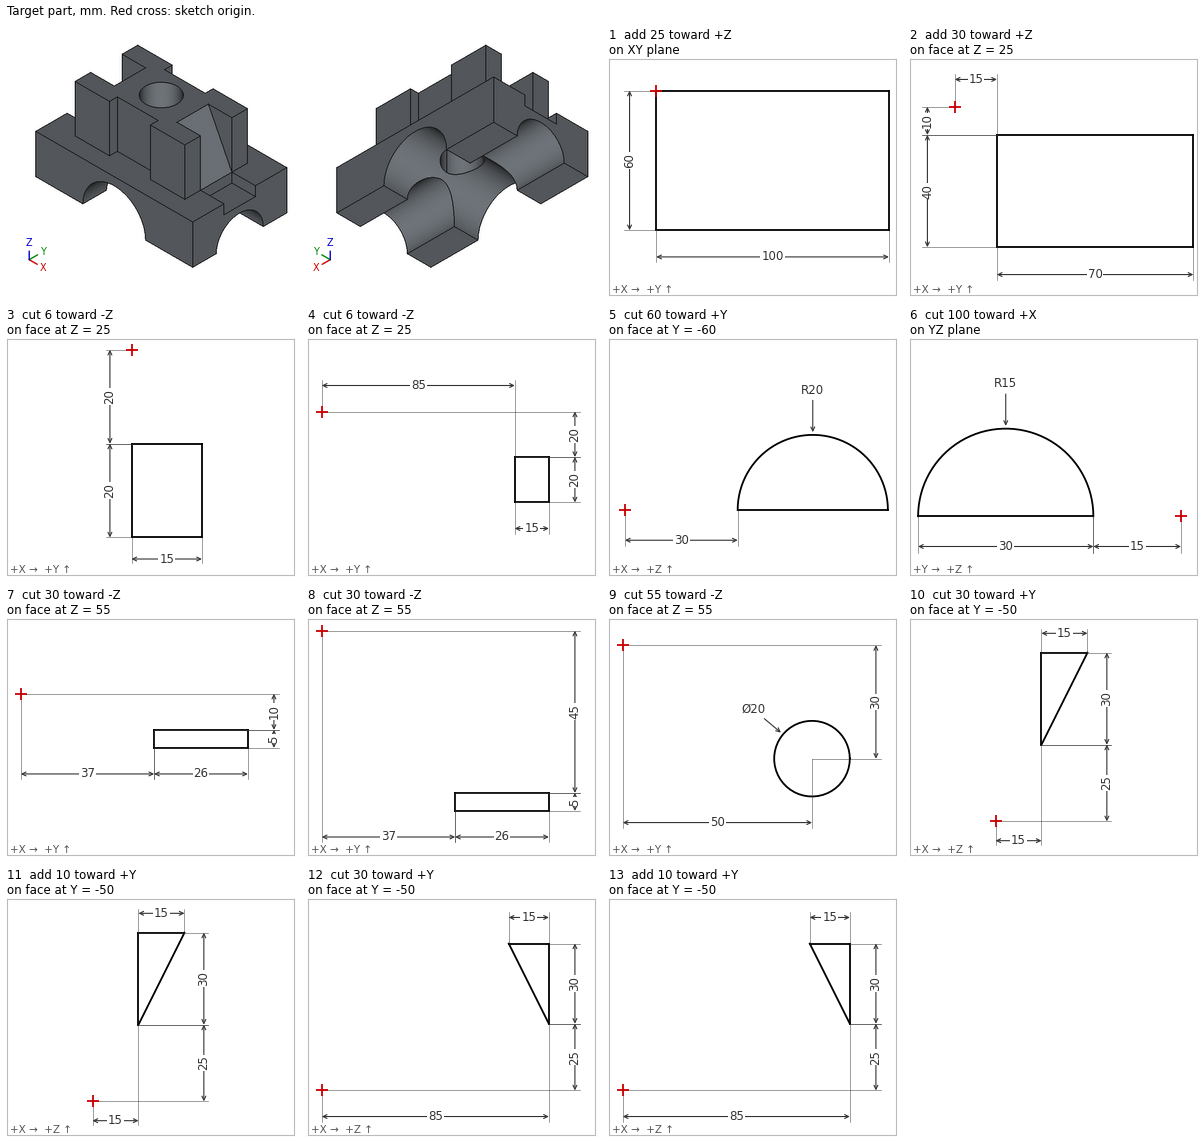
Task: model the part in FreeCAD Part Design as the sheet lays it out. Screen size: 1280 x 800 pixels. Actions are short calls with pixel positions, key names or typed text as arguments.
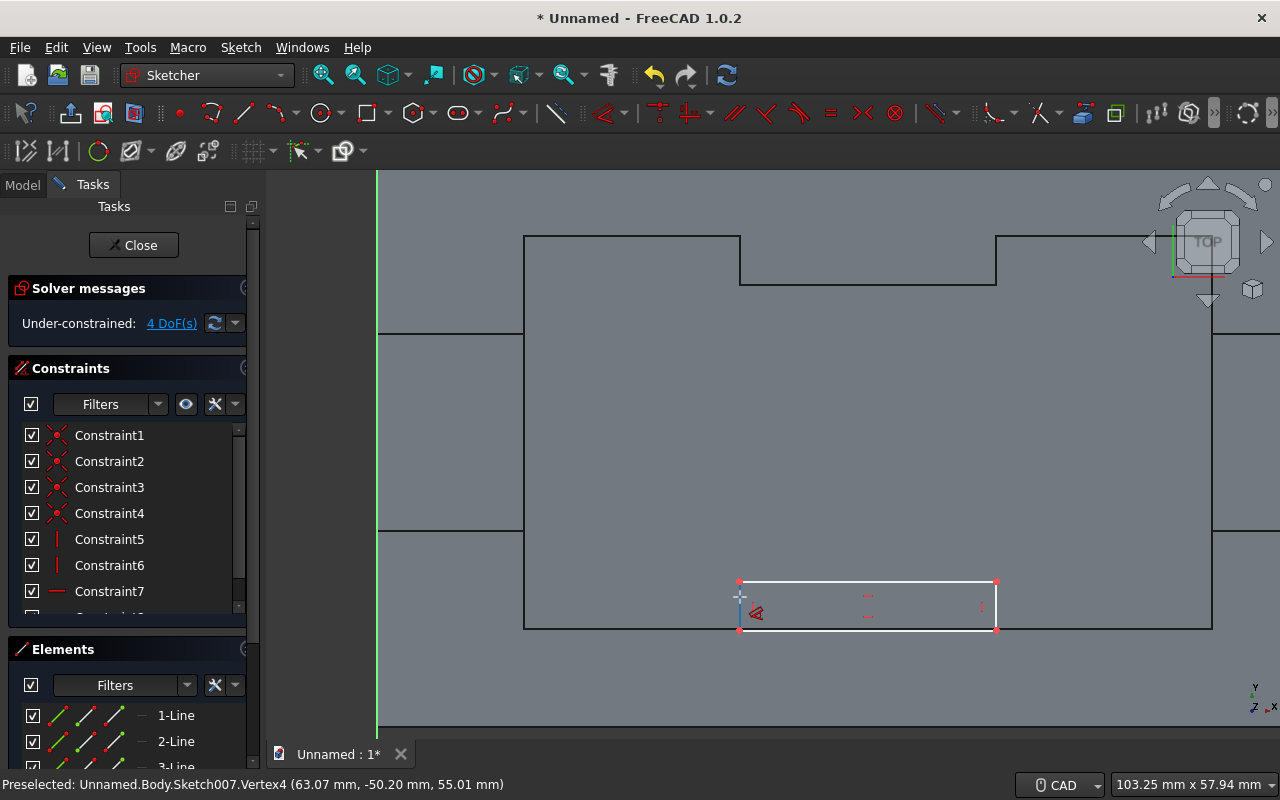
click(740, 596)
click(774, 606)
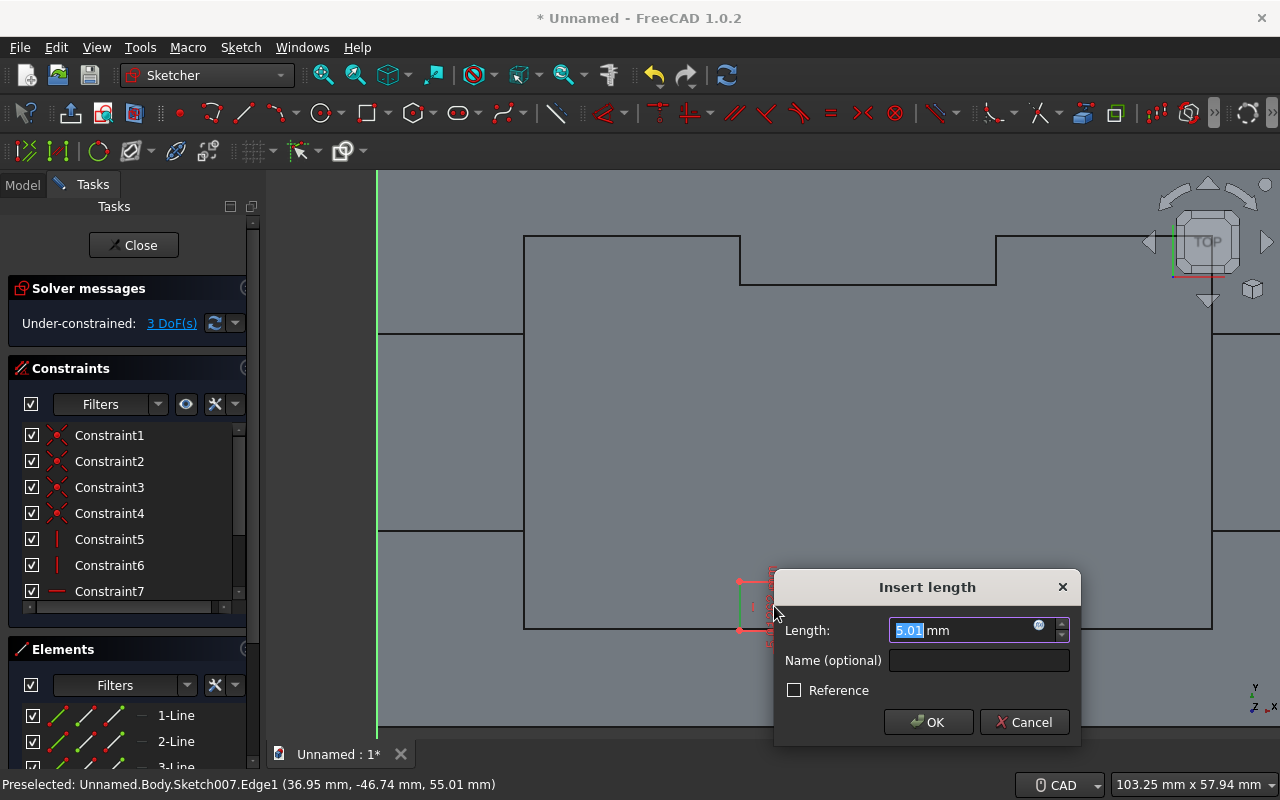
text(5)
key(Return)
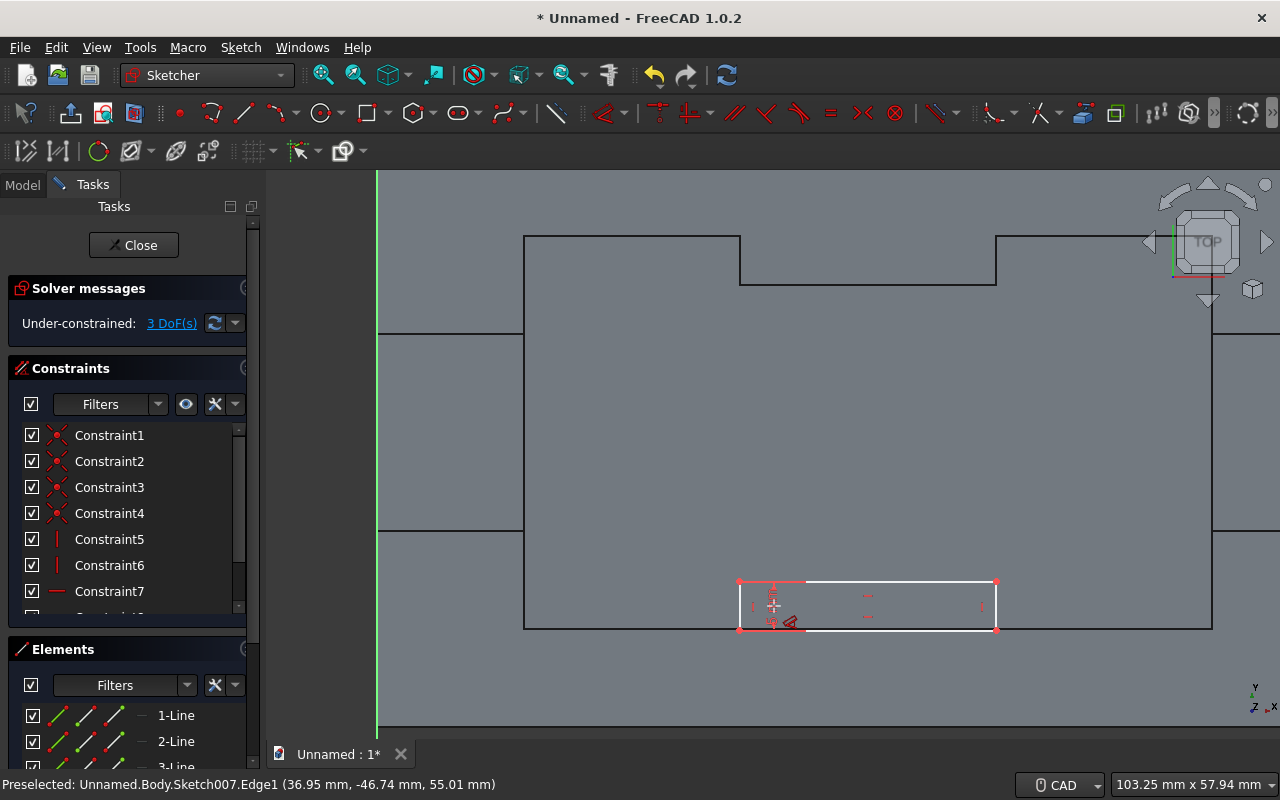
click(817, 631)
click(868, 665)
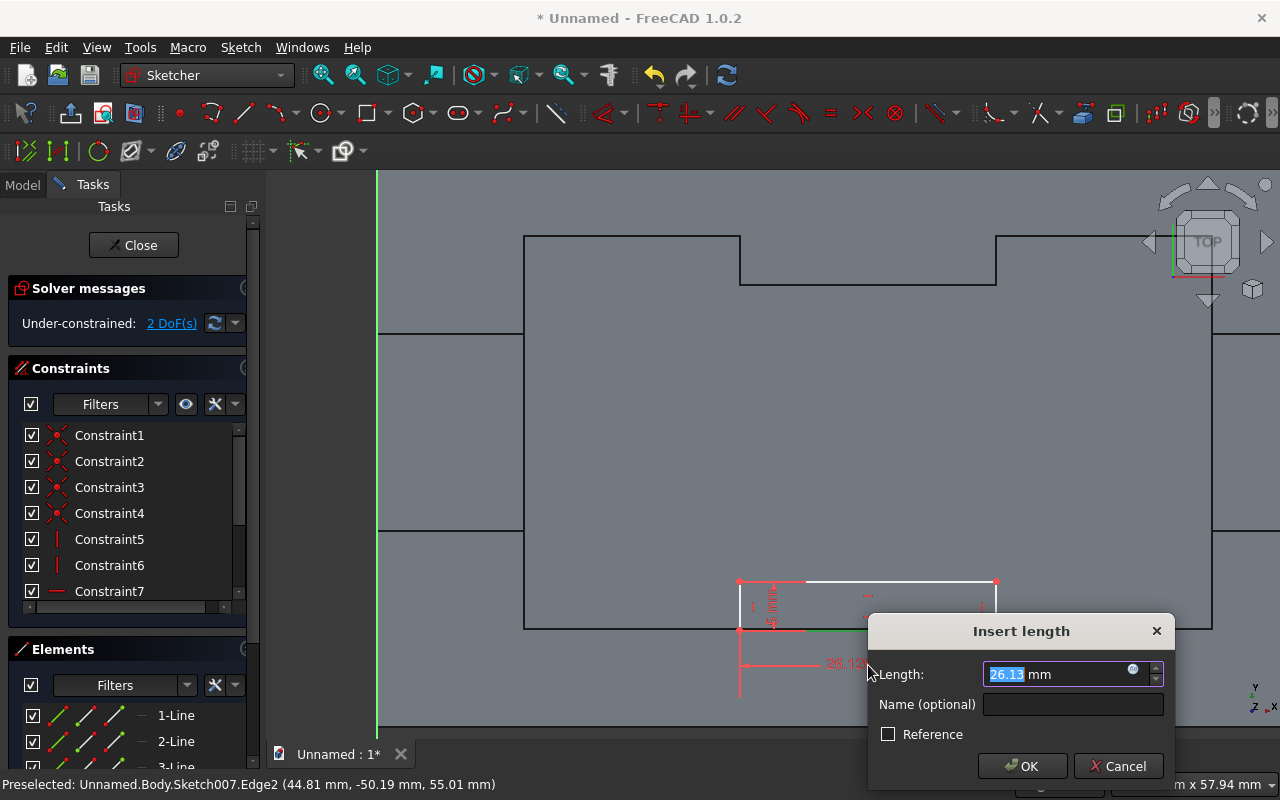
text(26)
key(Return)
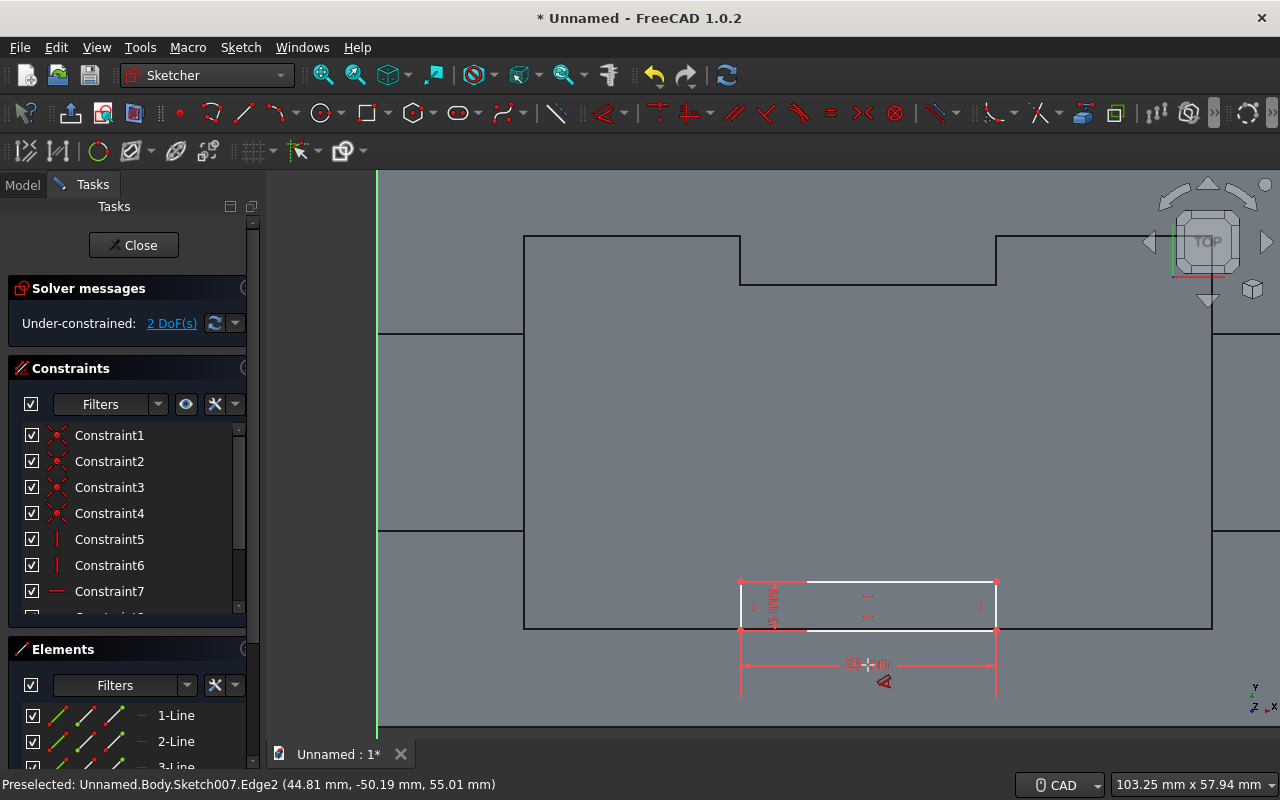
click(741, 582)
click(559, 616)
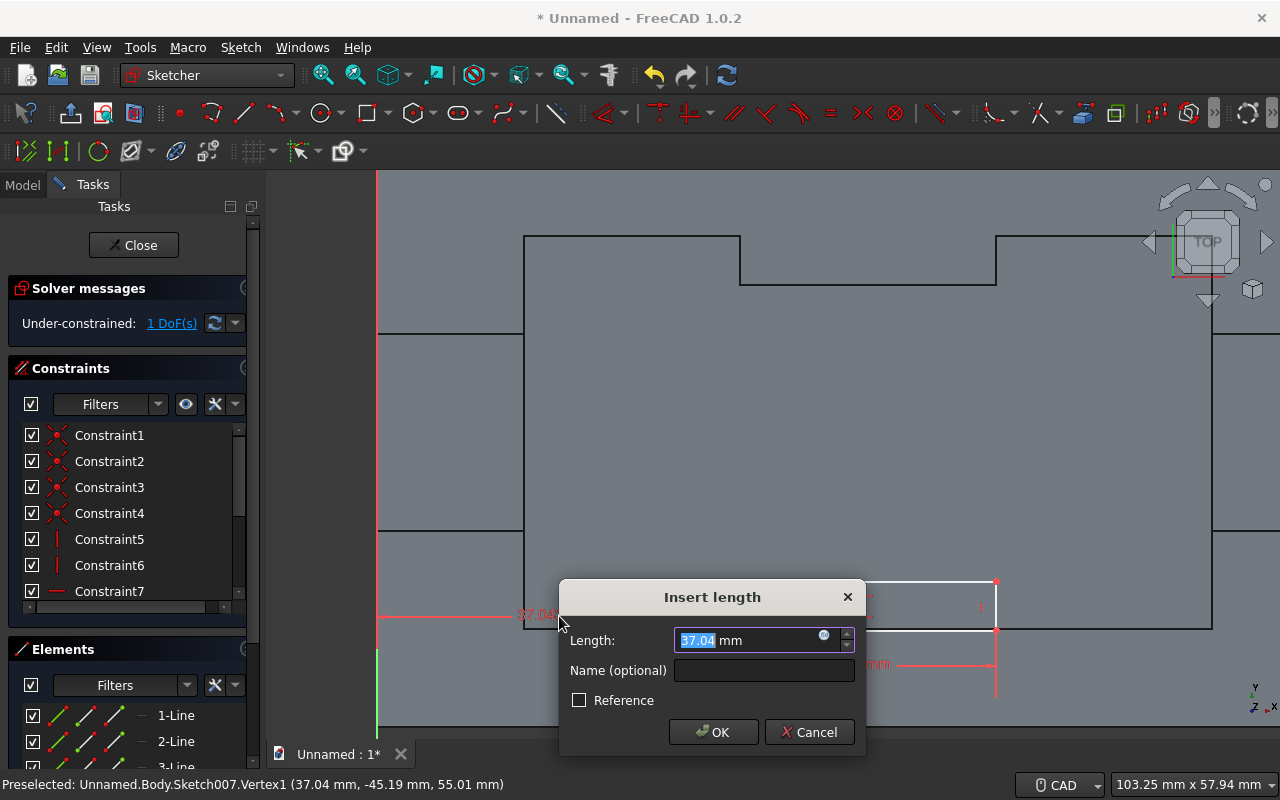
text(37)
key(Return)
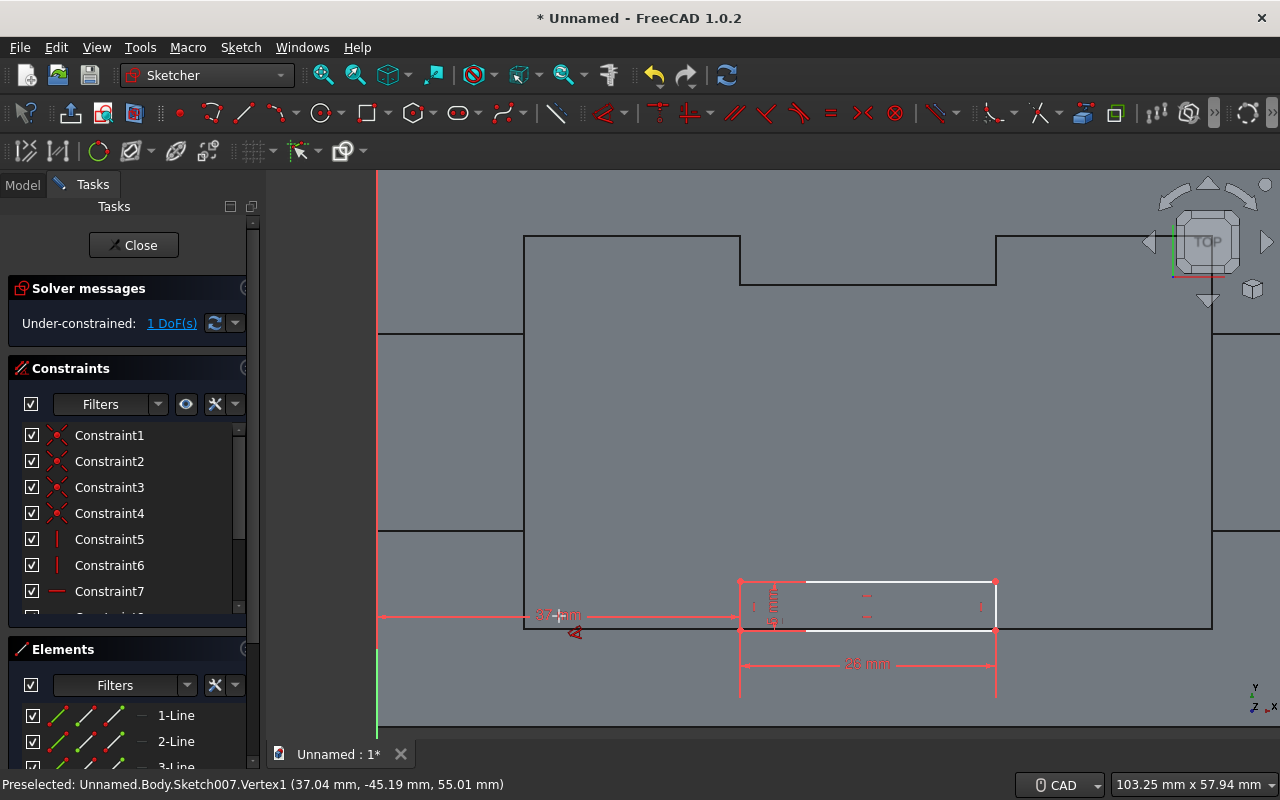
click(740, 582)
click(343, 390)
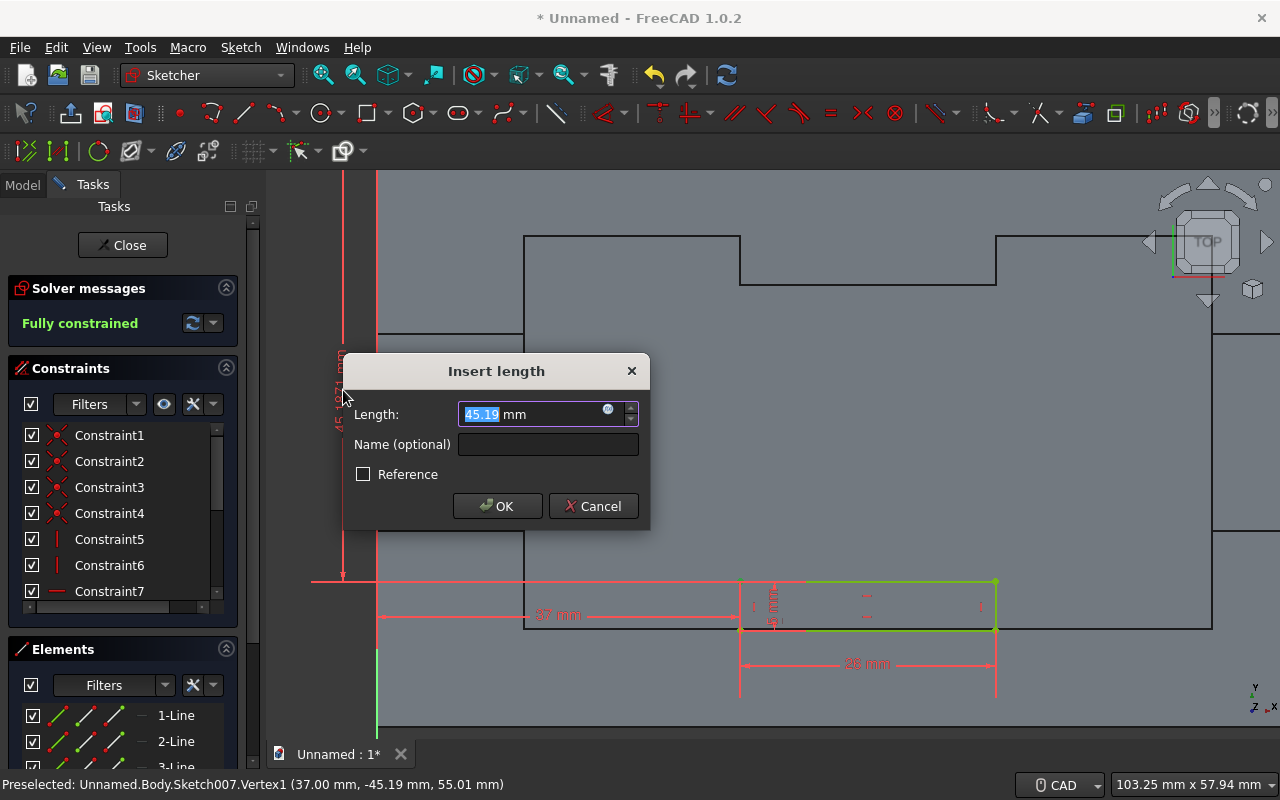
text(45)
key(Return)
key(Escape)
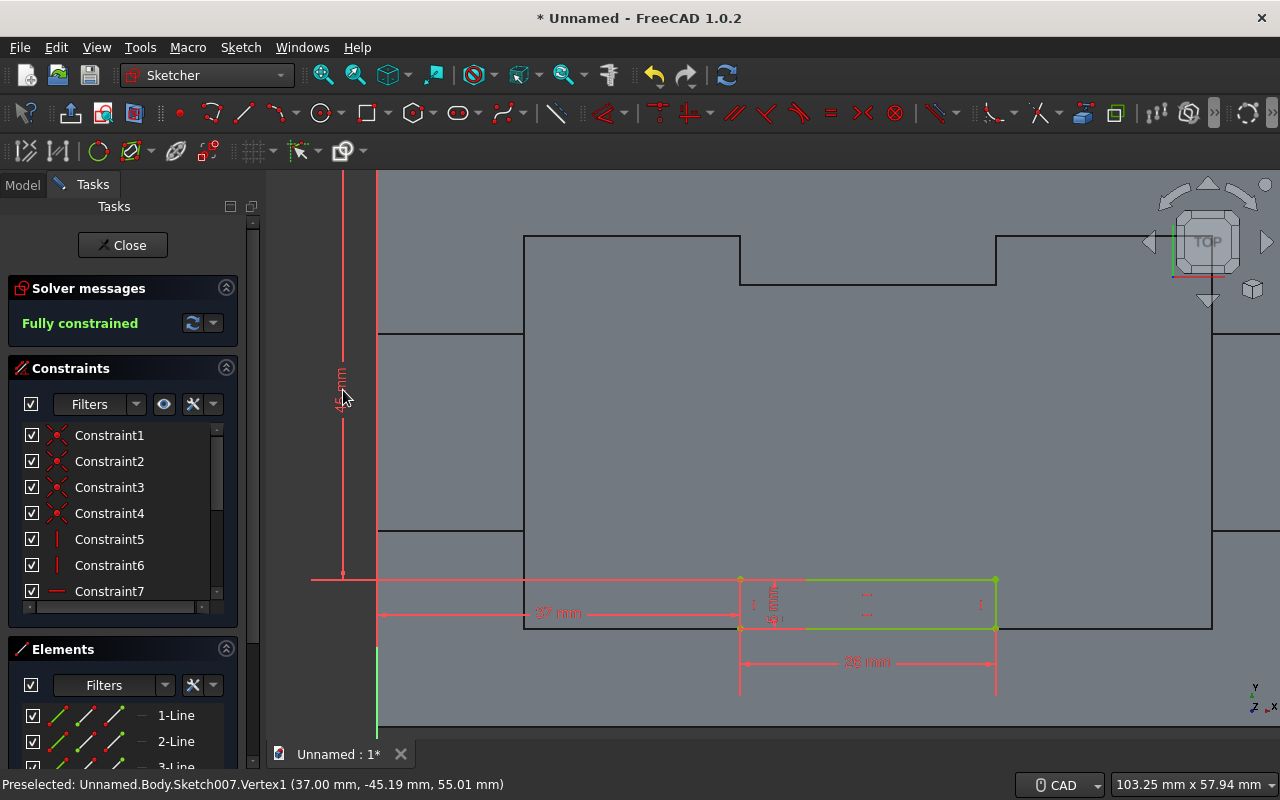
click(123, 245)